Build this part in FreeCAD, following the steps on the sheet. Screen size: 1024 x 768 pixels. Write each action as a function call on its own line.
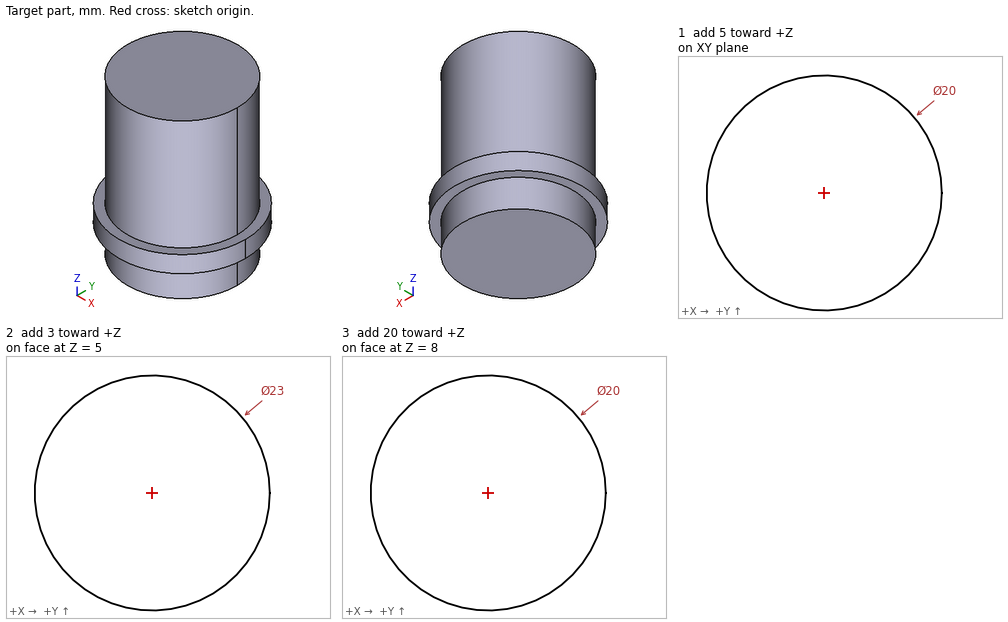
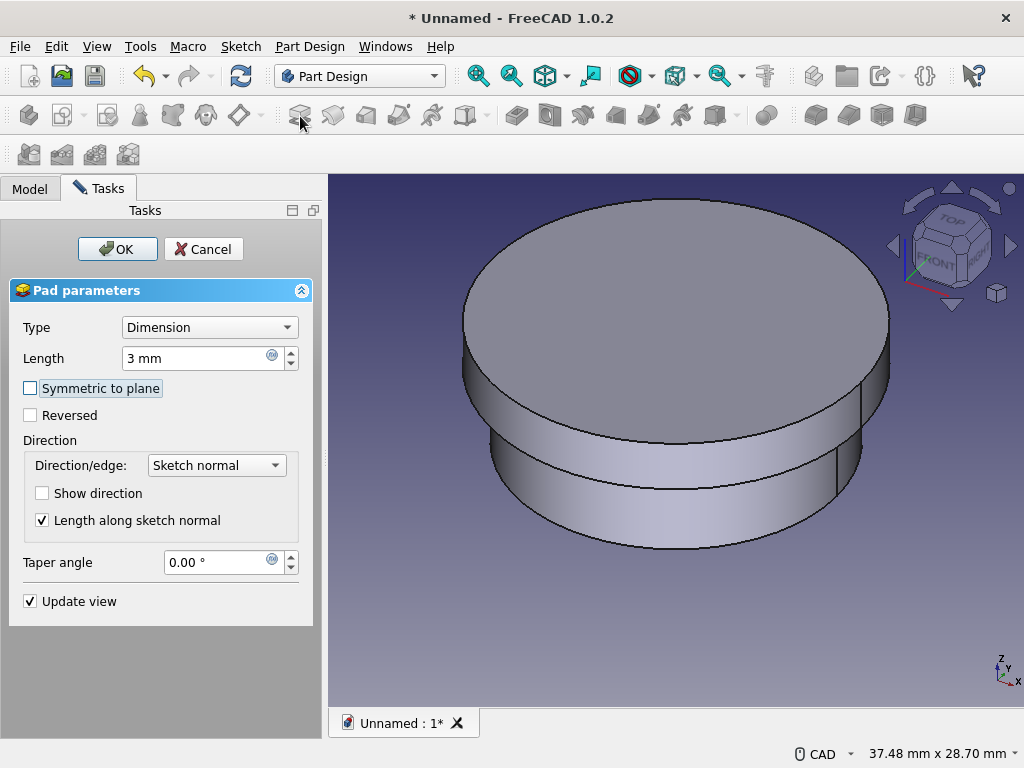
click(118, 249)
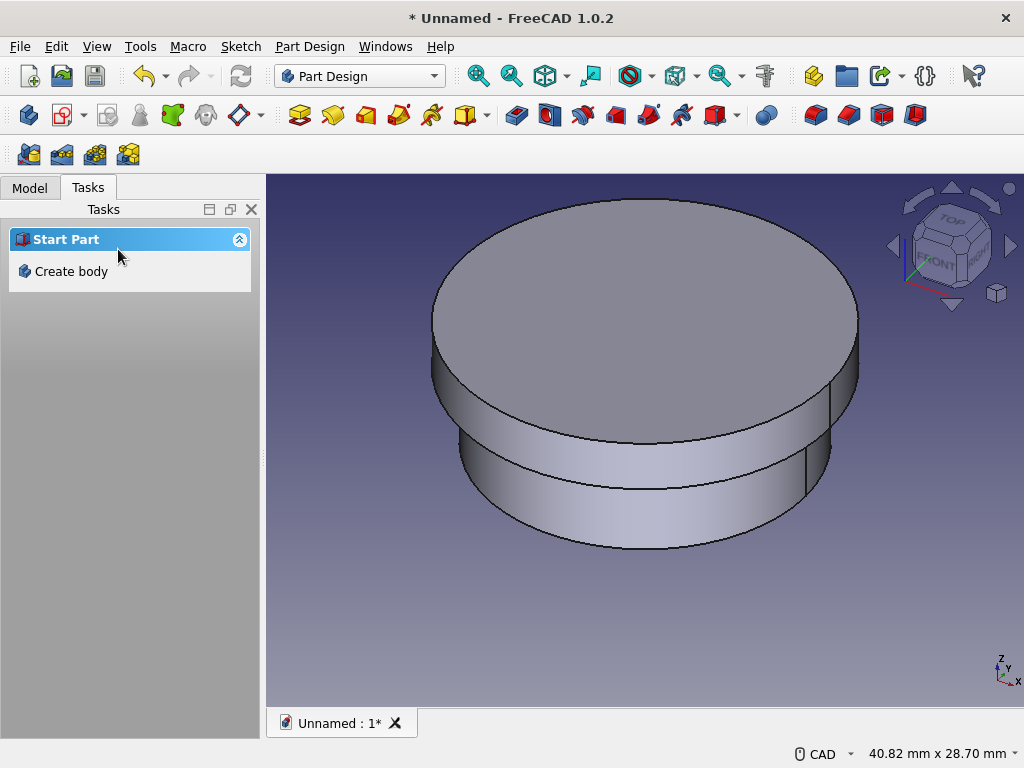
click(479, 76)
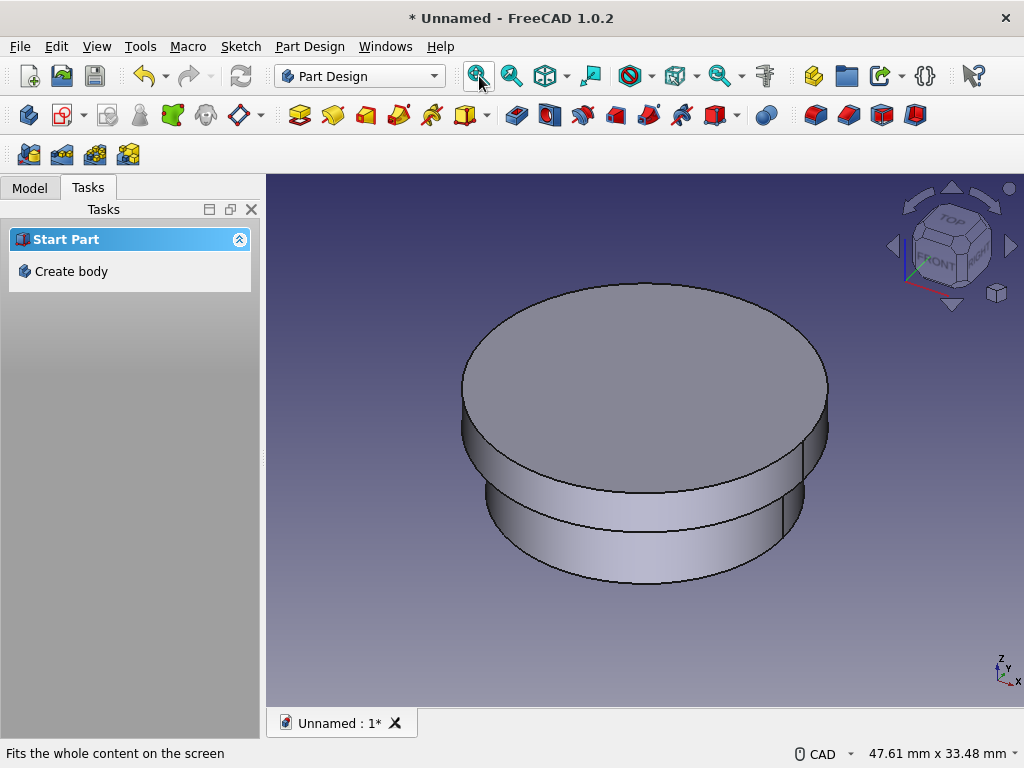
click(645, 387)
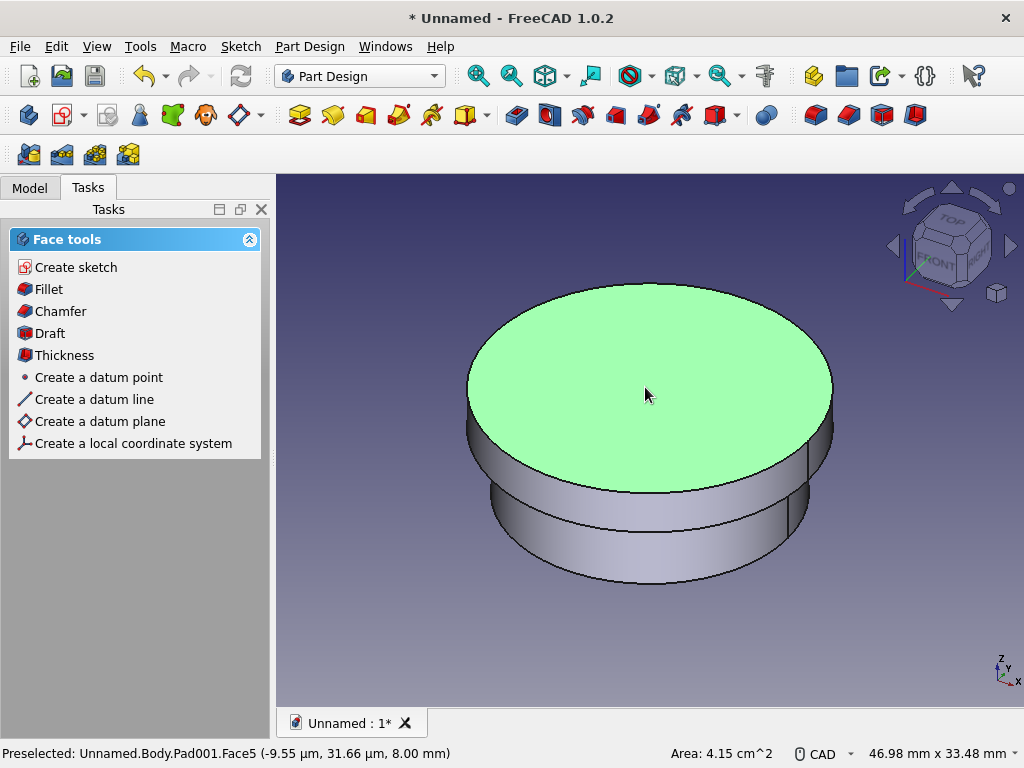
click(62, 116)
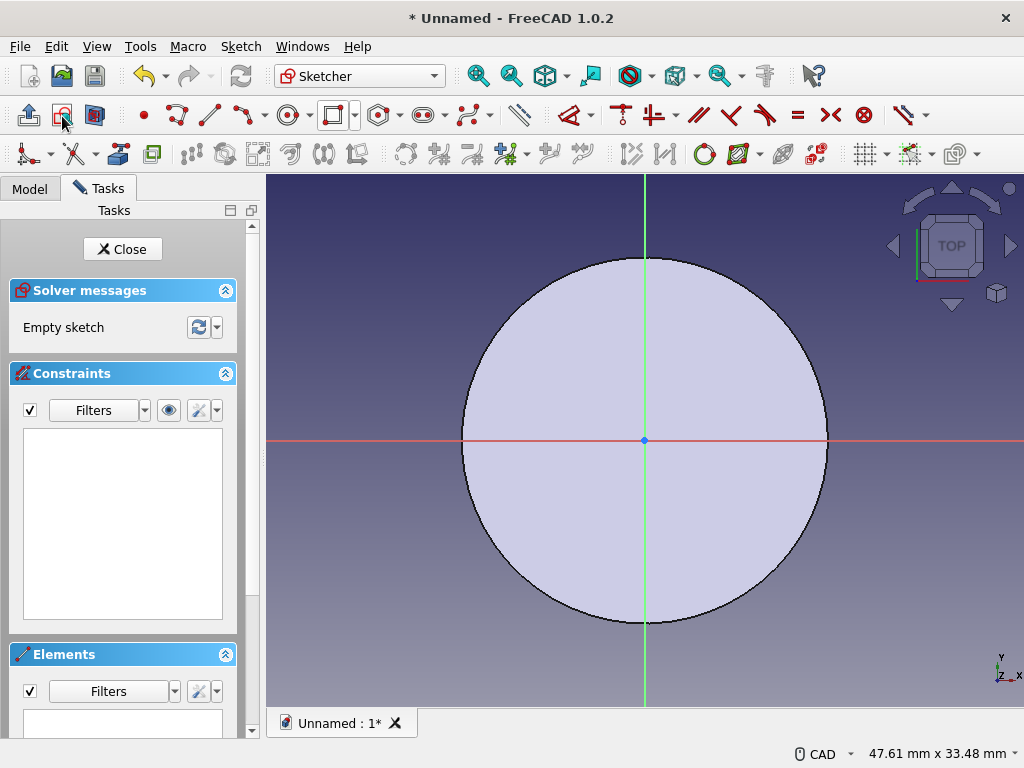
key(g)
key(c)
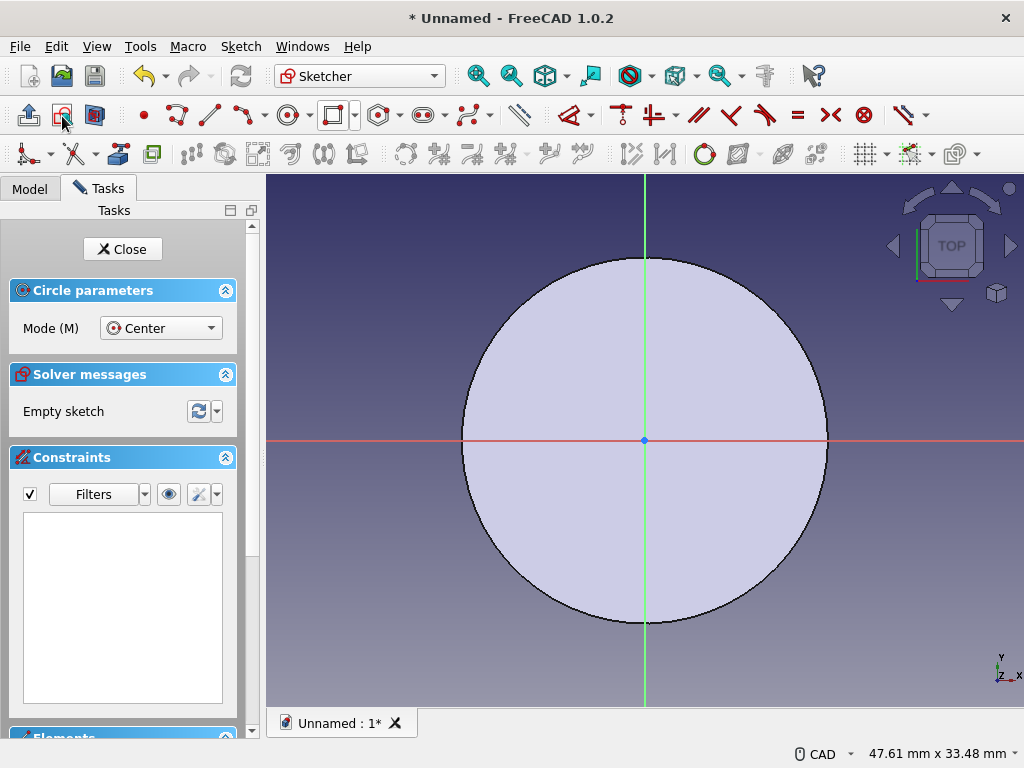
click(645, 440)
click(757, 328)
key(Escape)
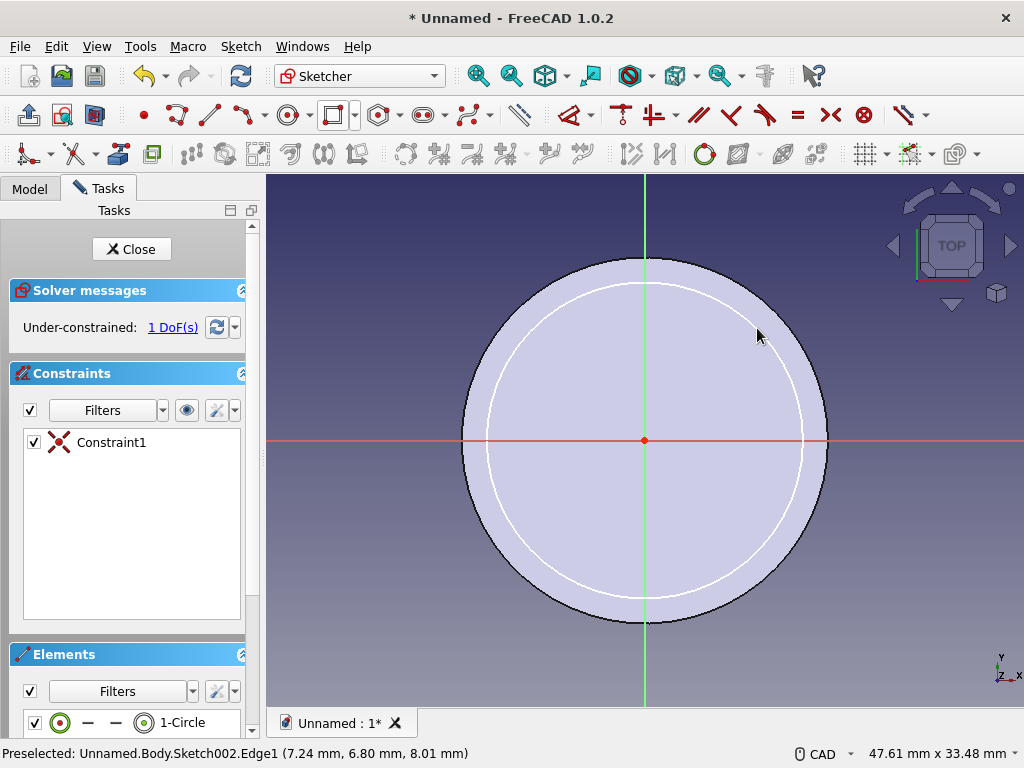
click(568, 116)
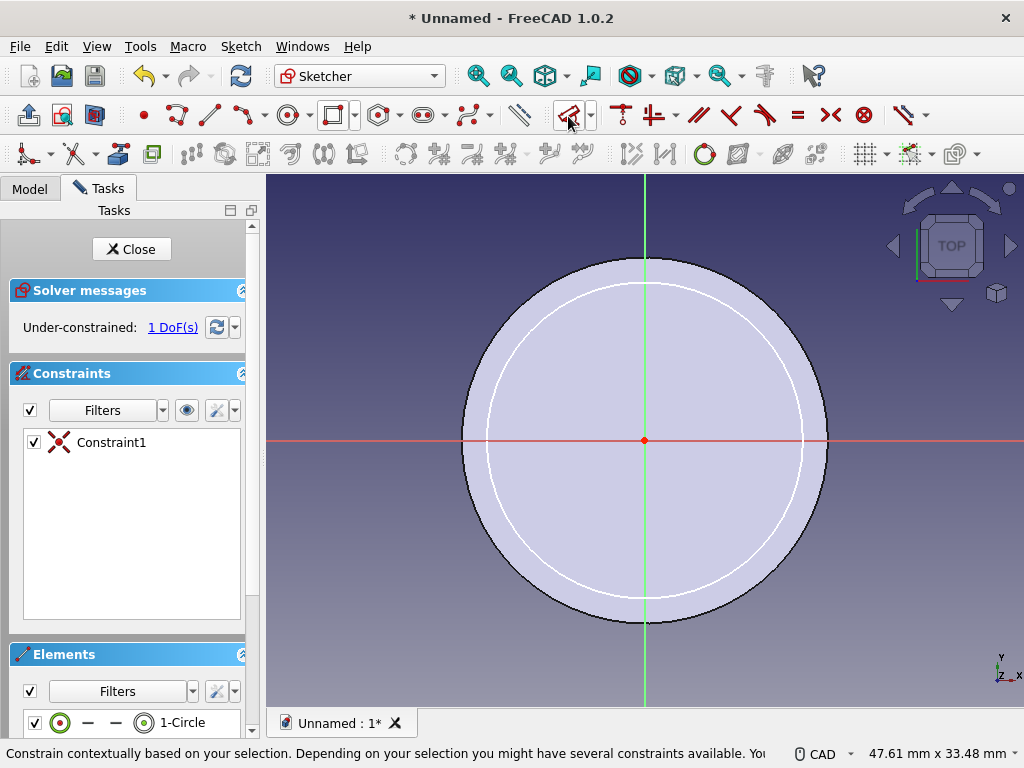
click(756, 328)
click(778, 305)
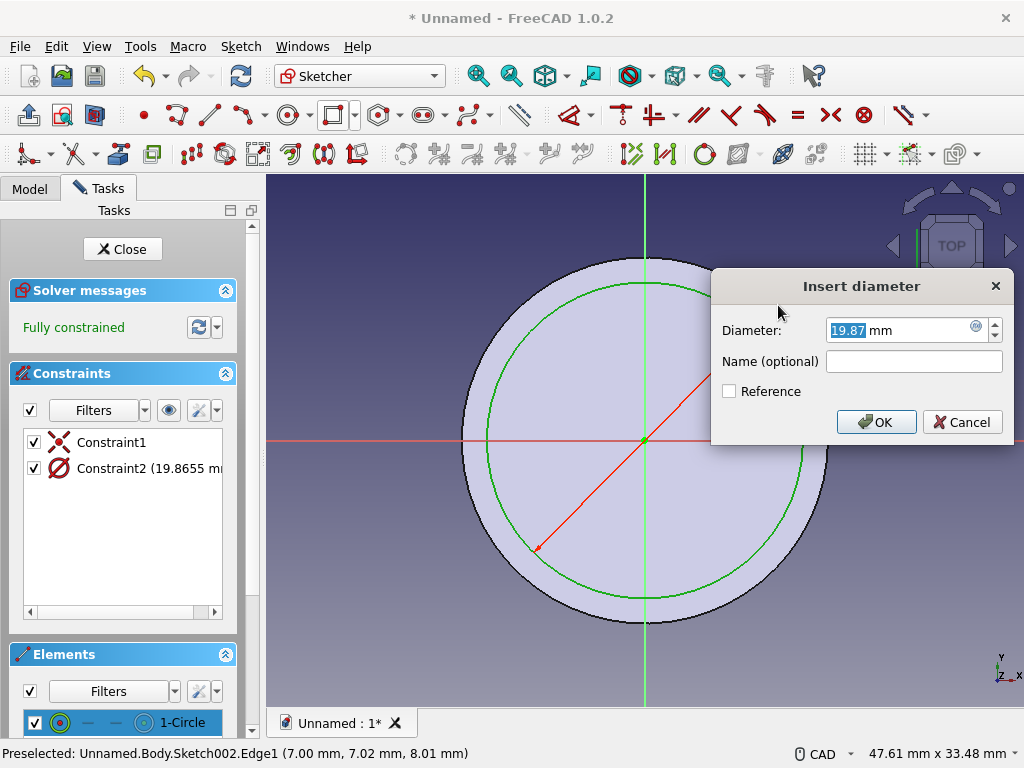
text(20)
key(Return)
key(Escape)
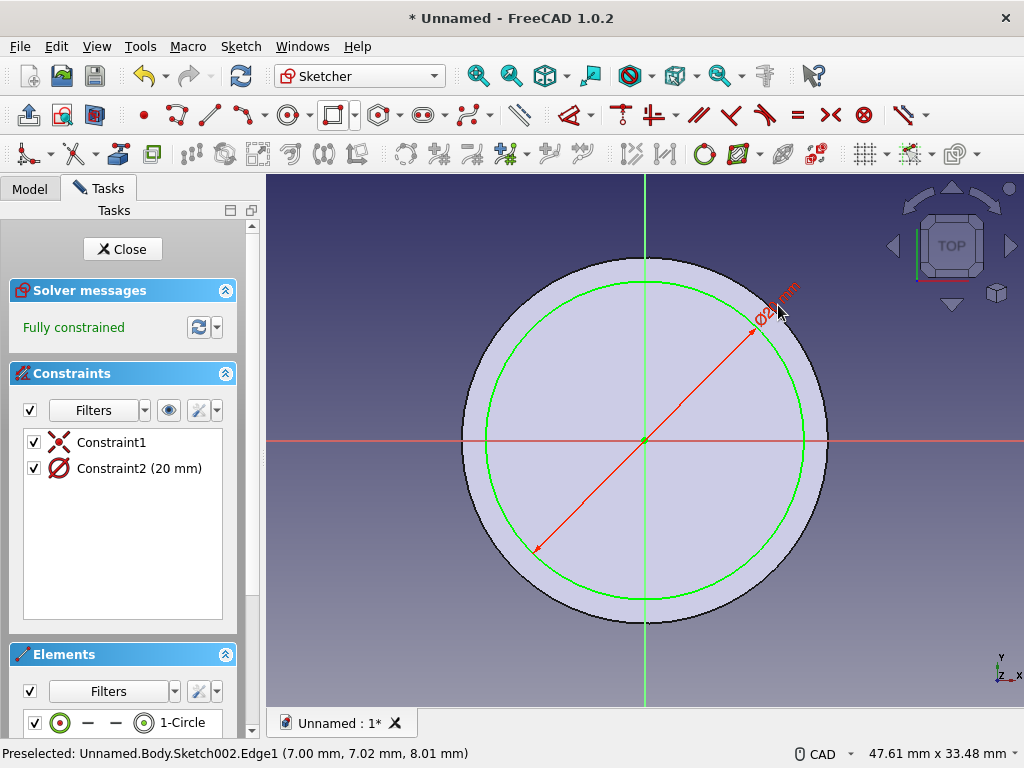
click(123, 249)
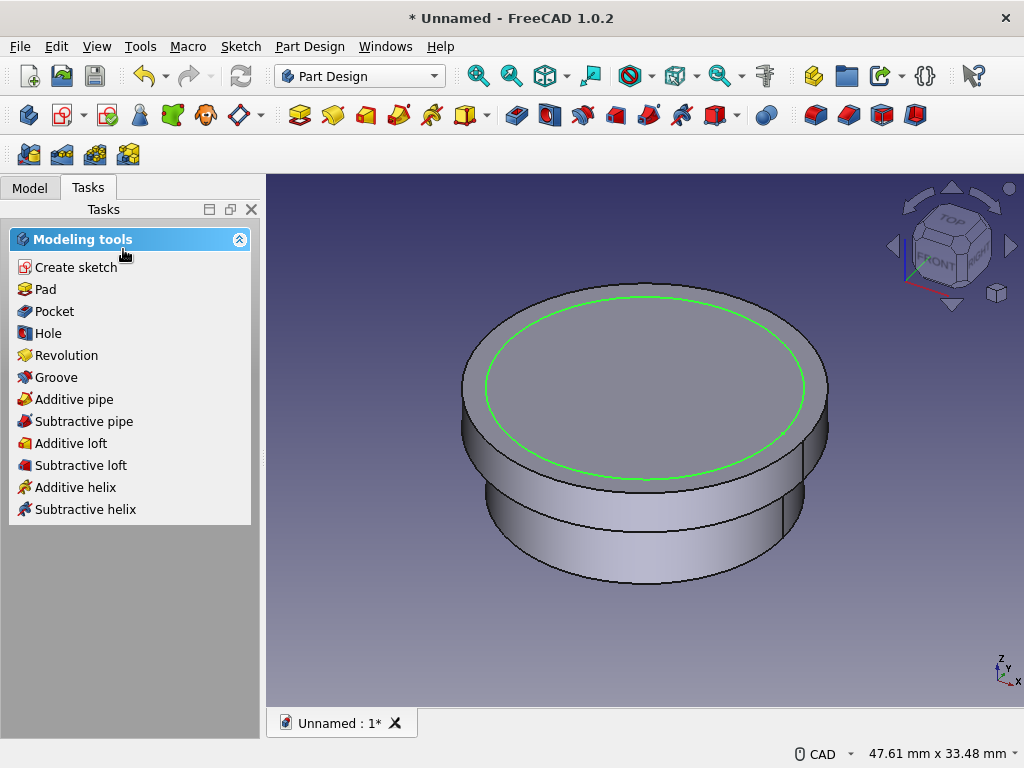
click(300, 116)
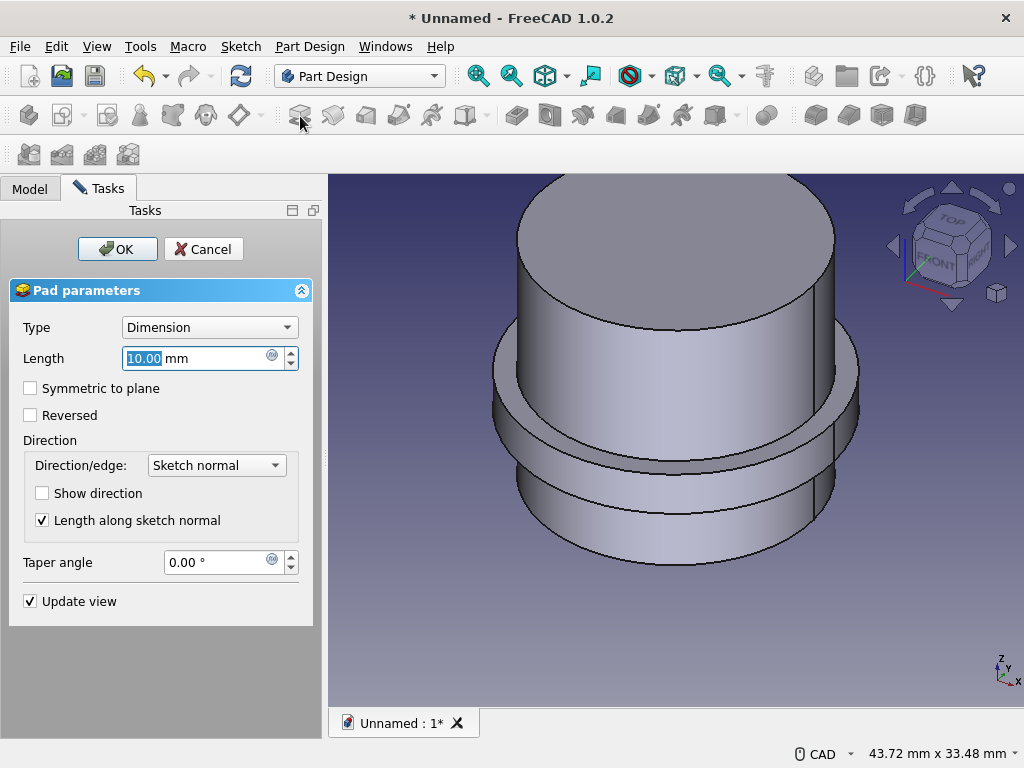
text(20)
key(Tab)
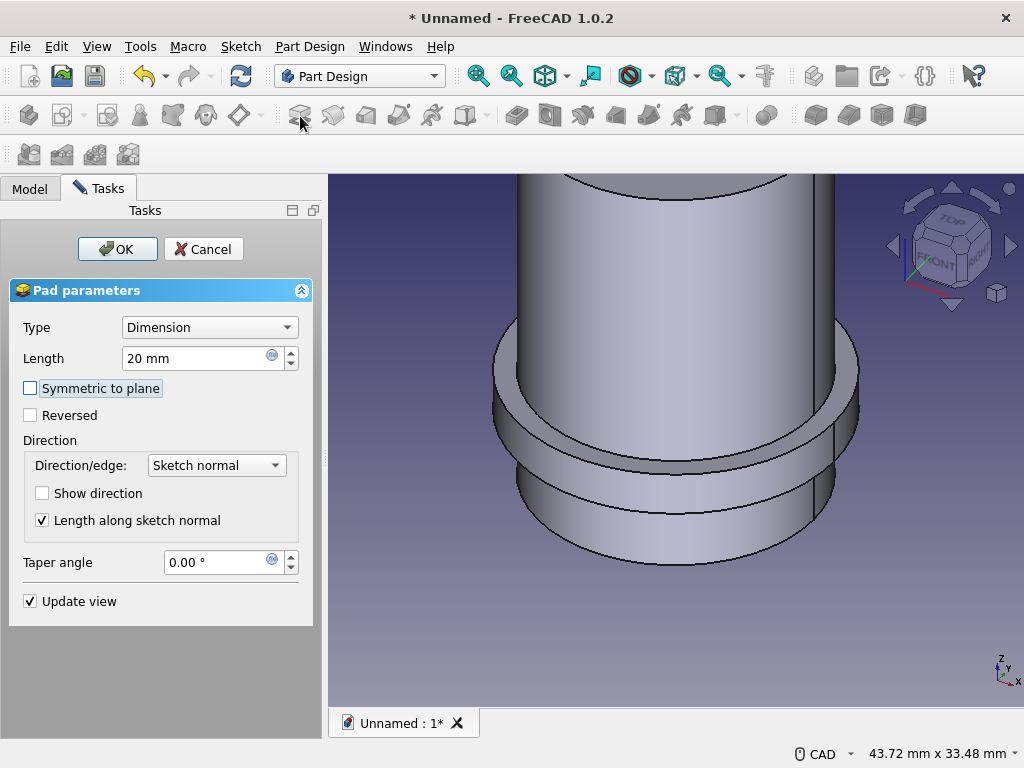
click(118, 249)